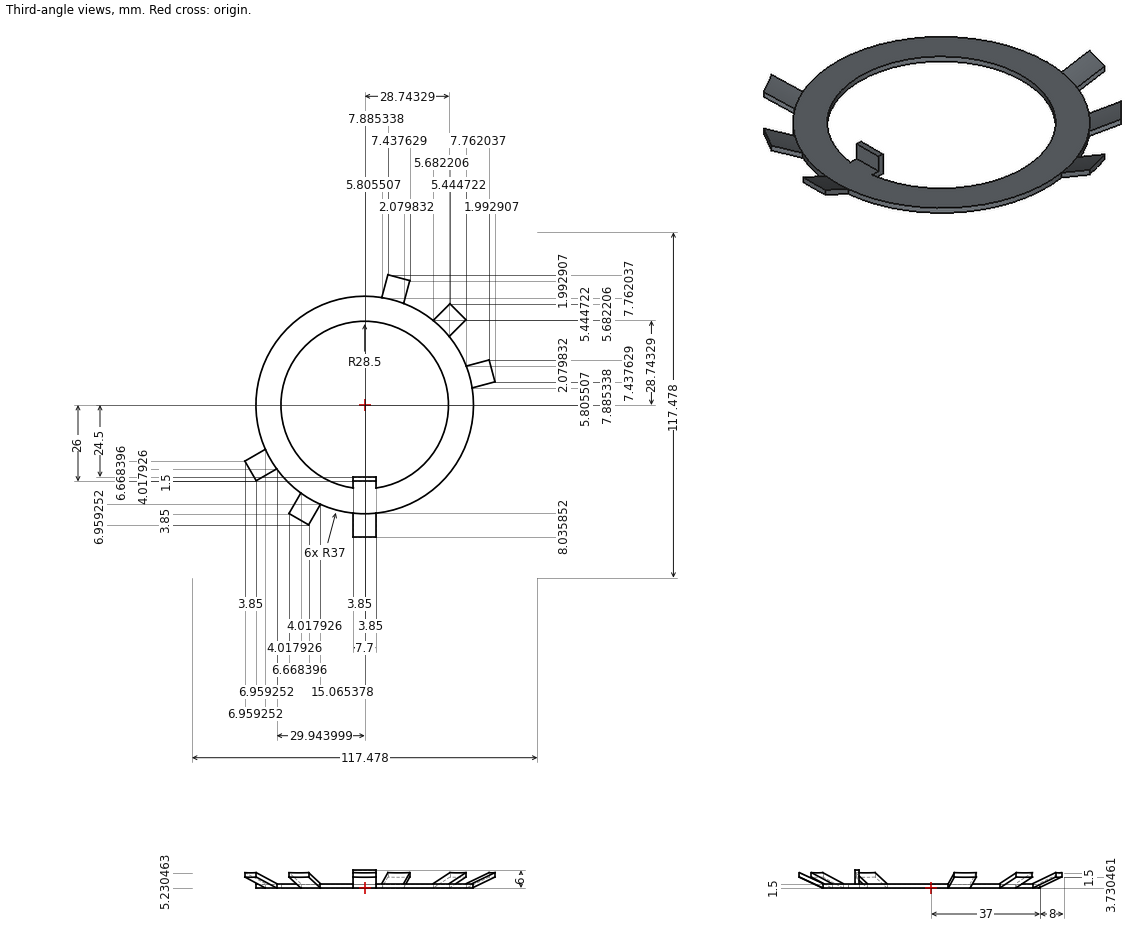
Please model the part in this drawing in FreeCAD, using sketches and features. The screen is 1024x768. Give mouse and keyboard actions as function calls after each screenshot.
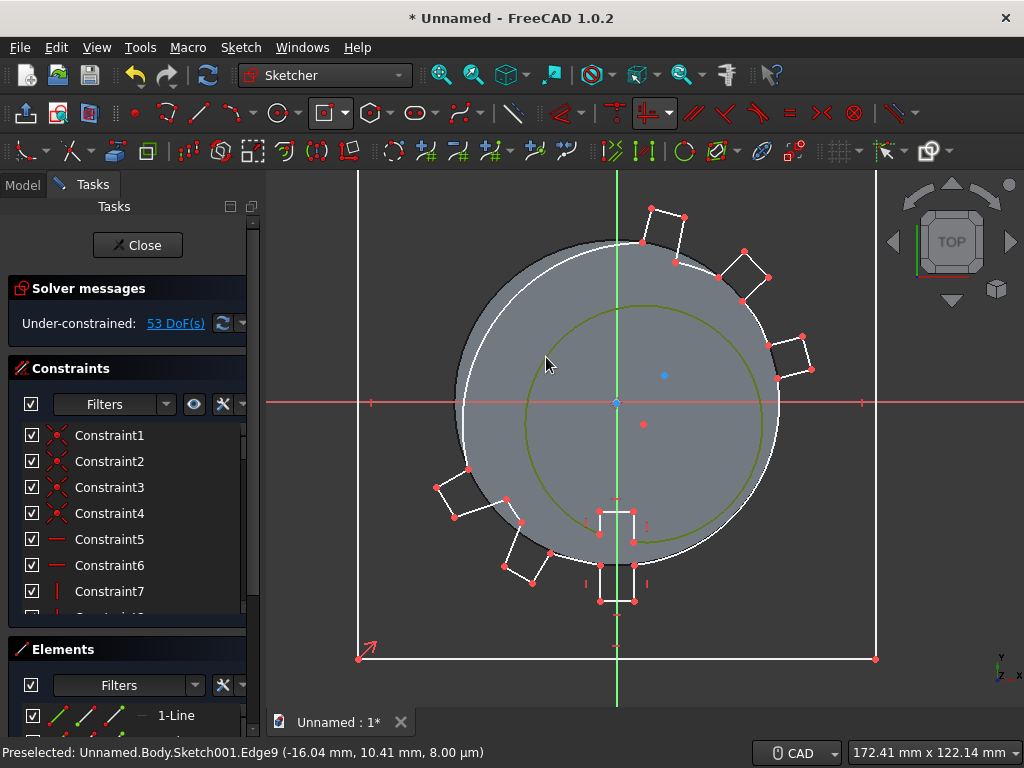
click(763, 331)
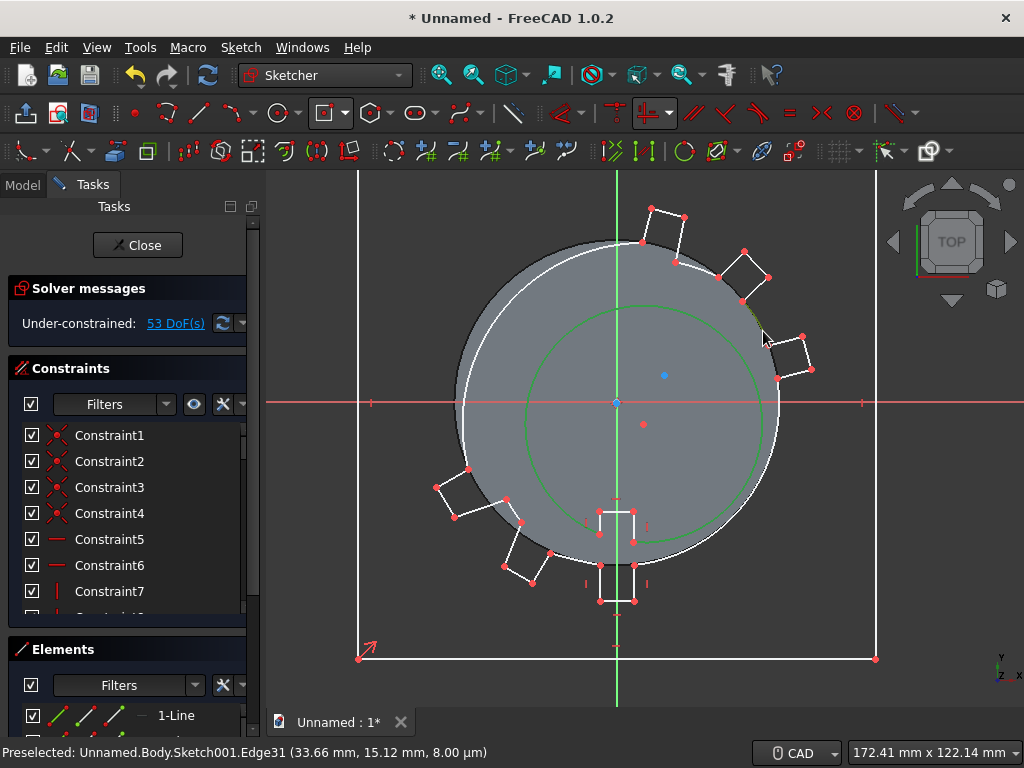
click(616, 114)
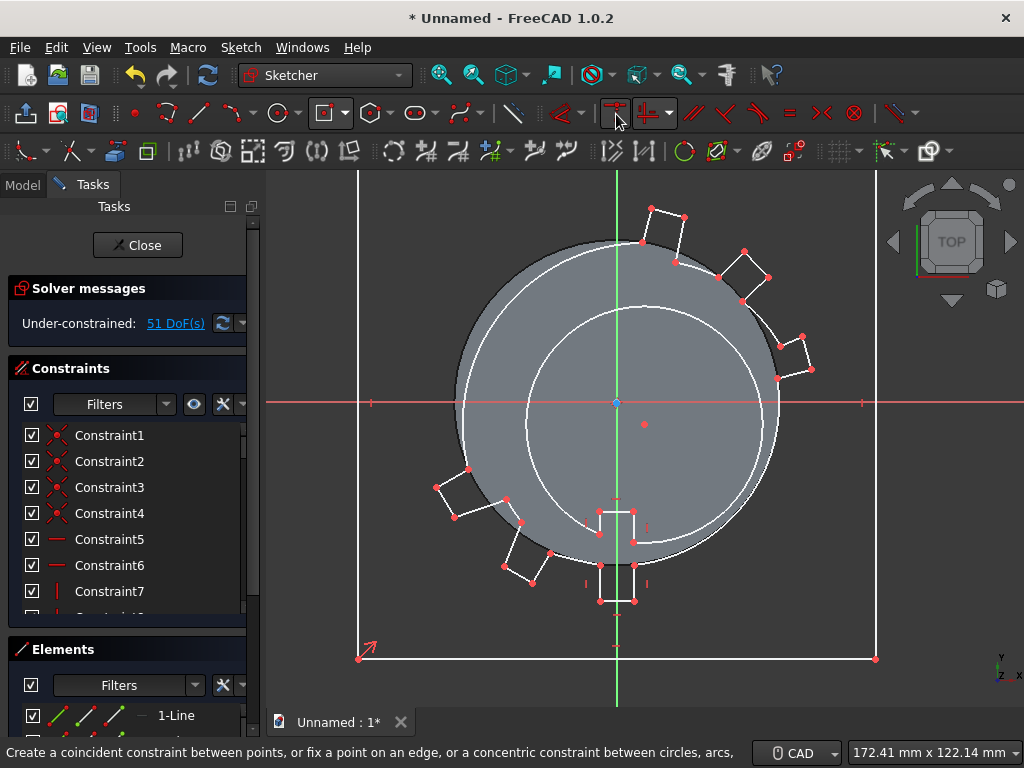
click(548, 357)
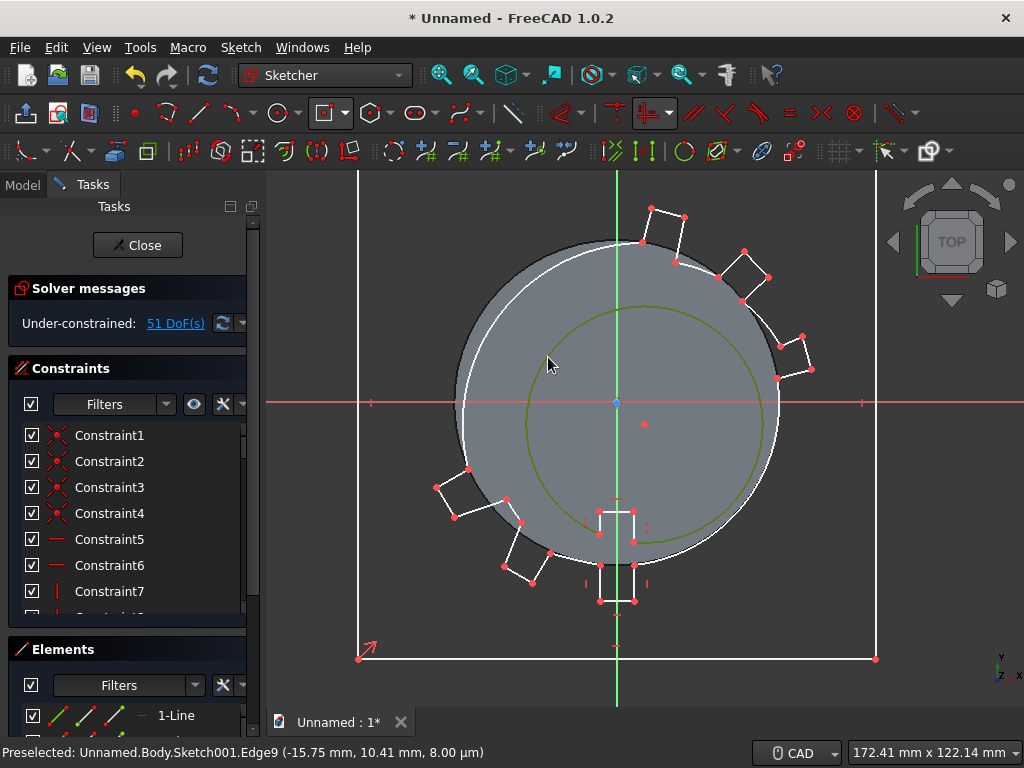
click(707, 538)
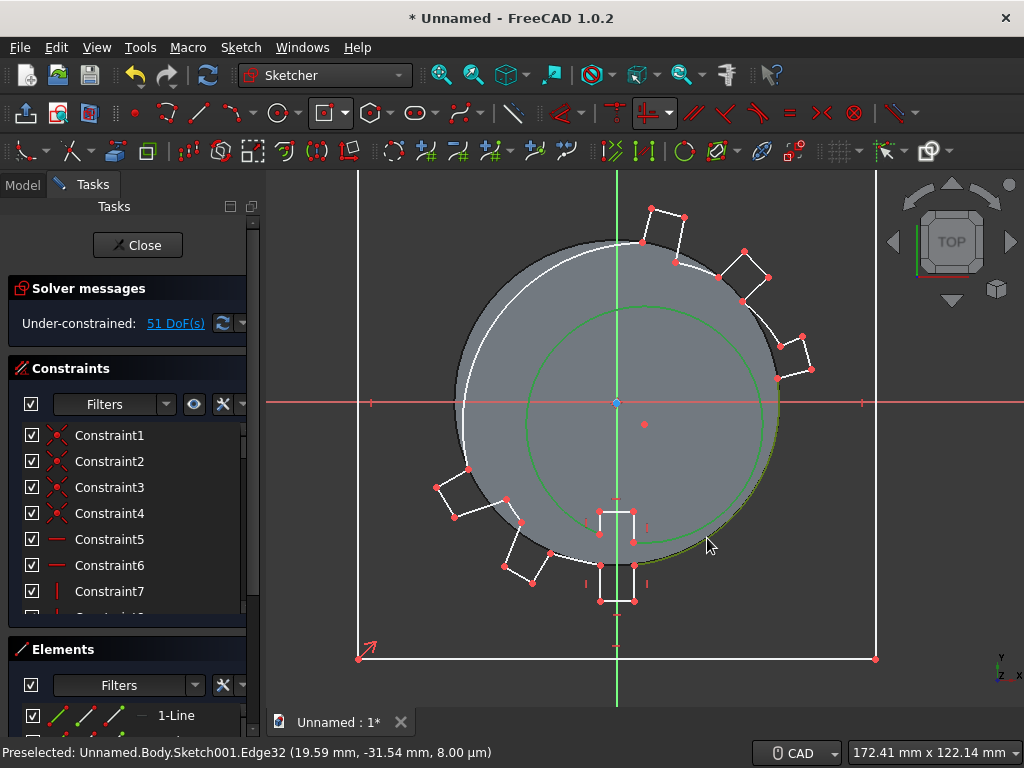
key(c)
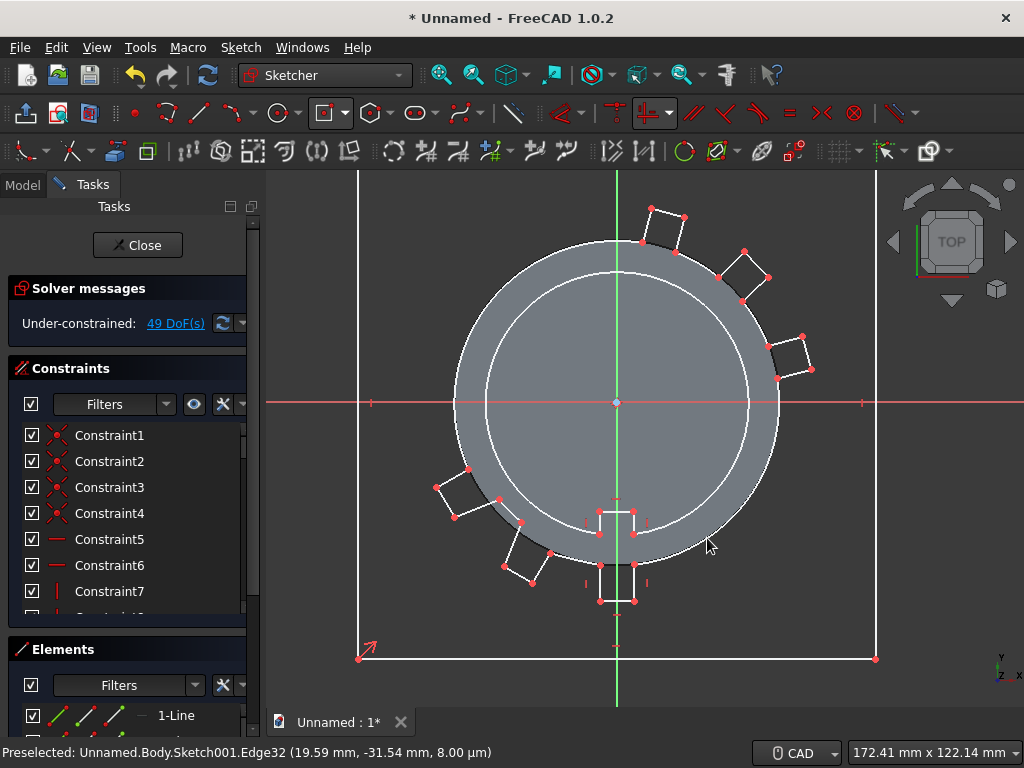
click(740, 357)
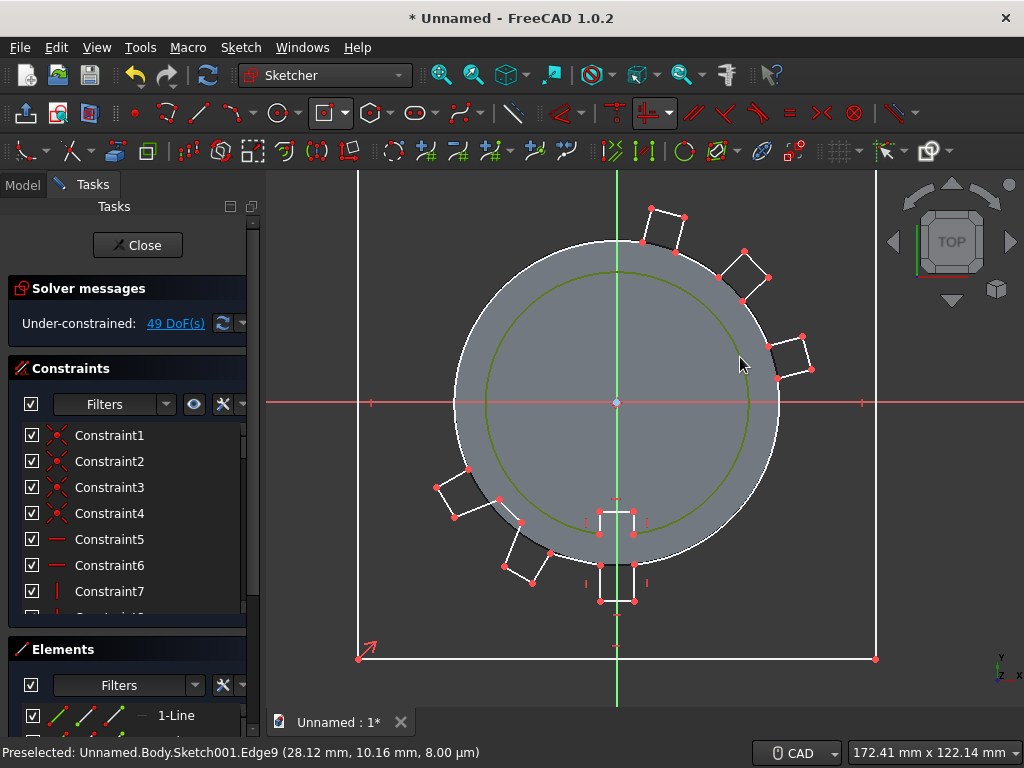
click(565, 557)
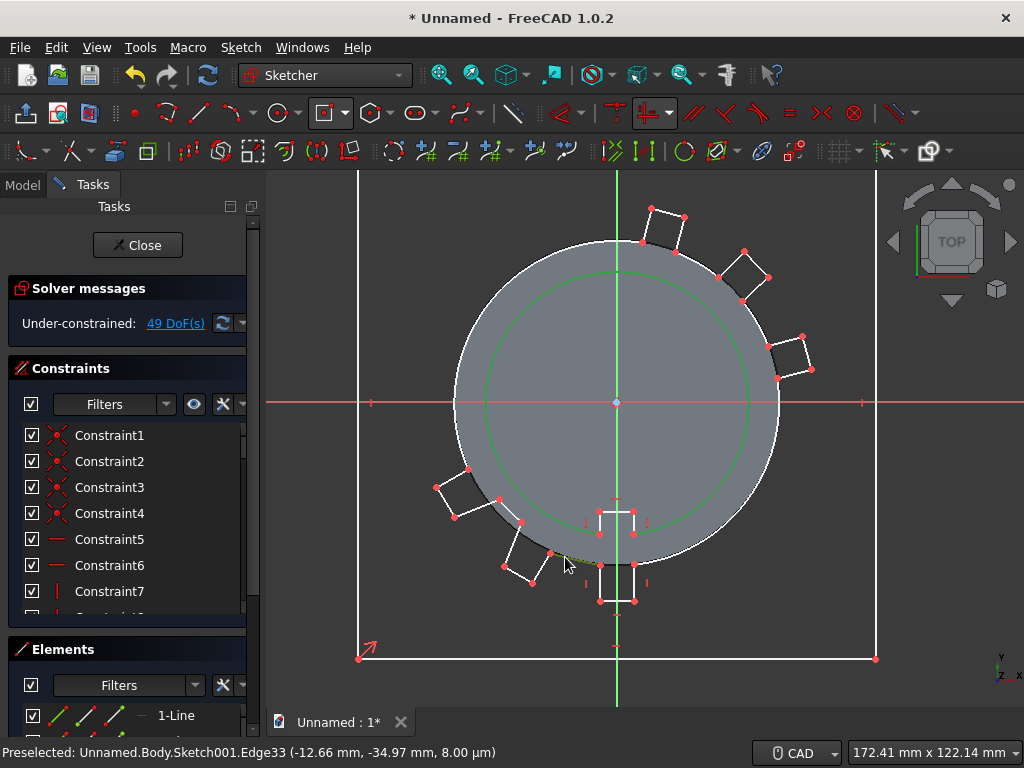
click(616, 114)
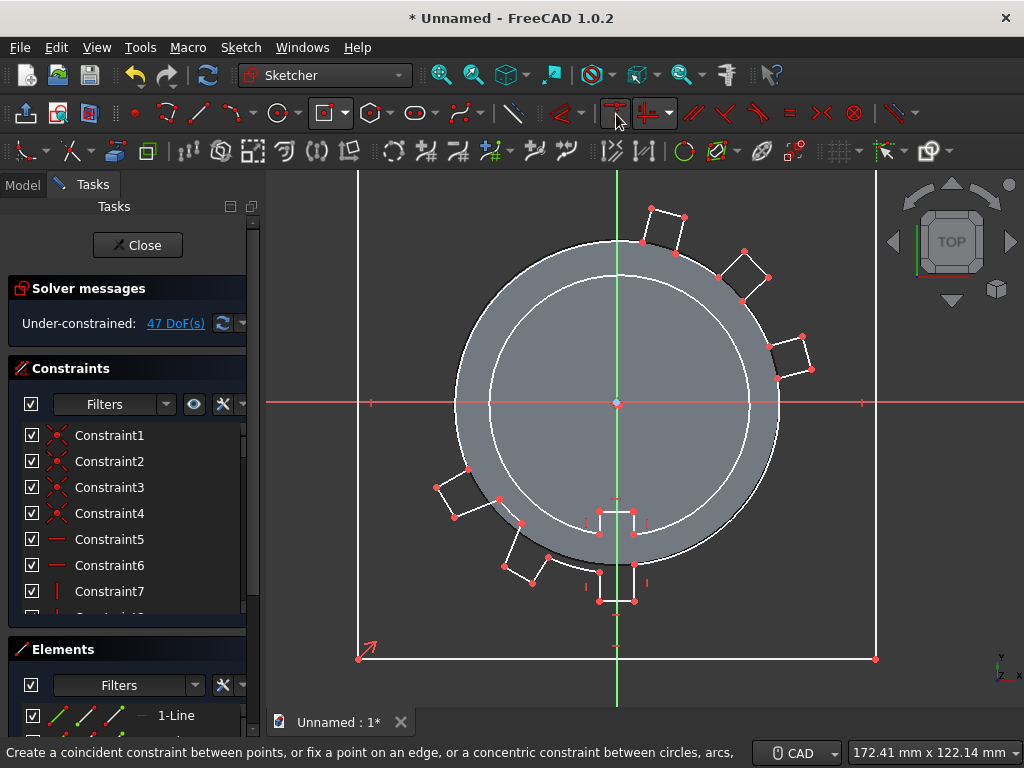
drag(607, 392, 630, 415)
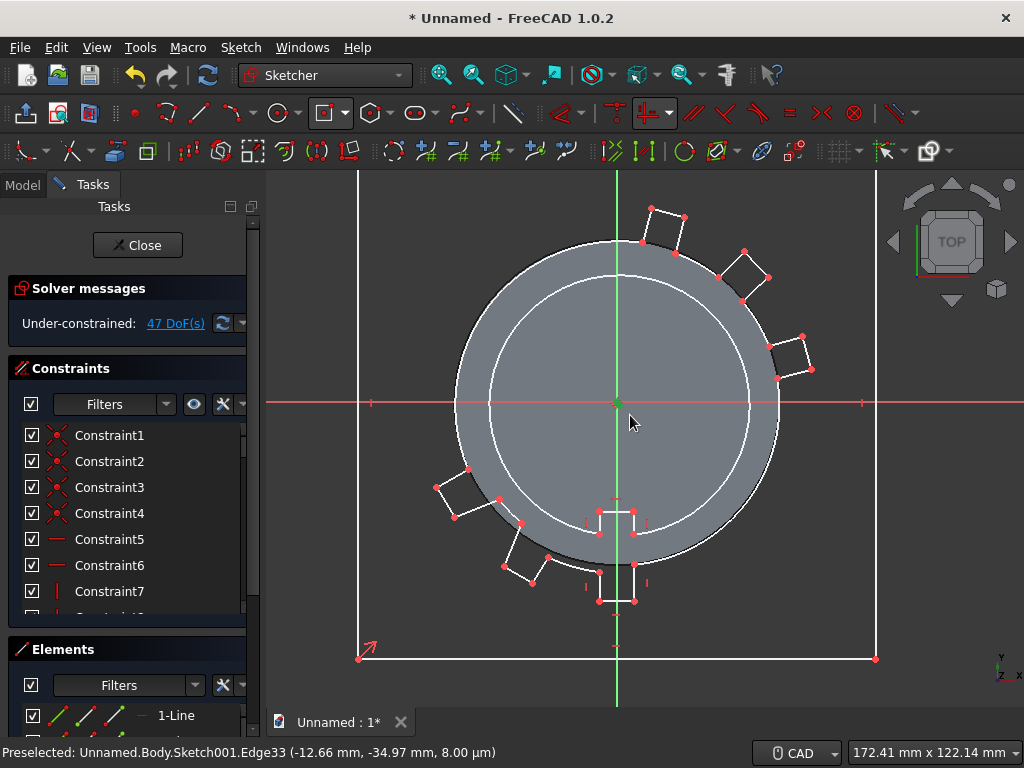
click(616, 114)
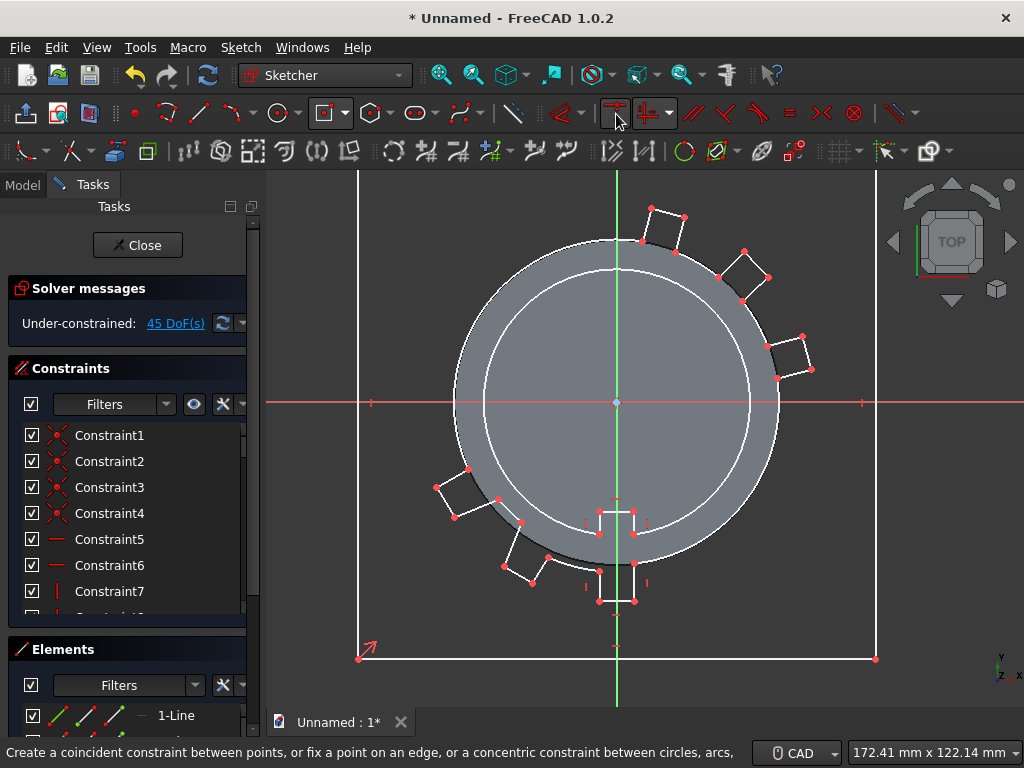
scroll(505, 507, up, 2)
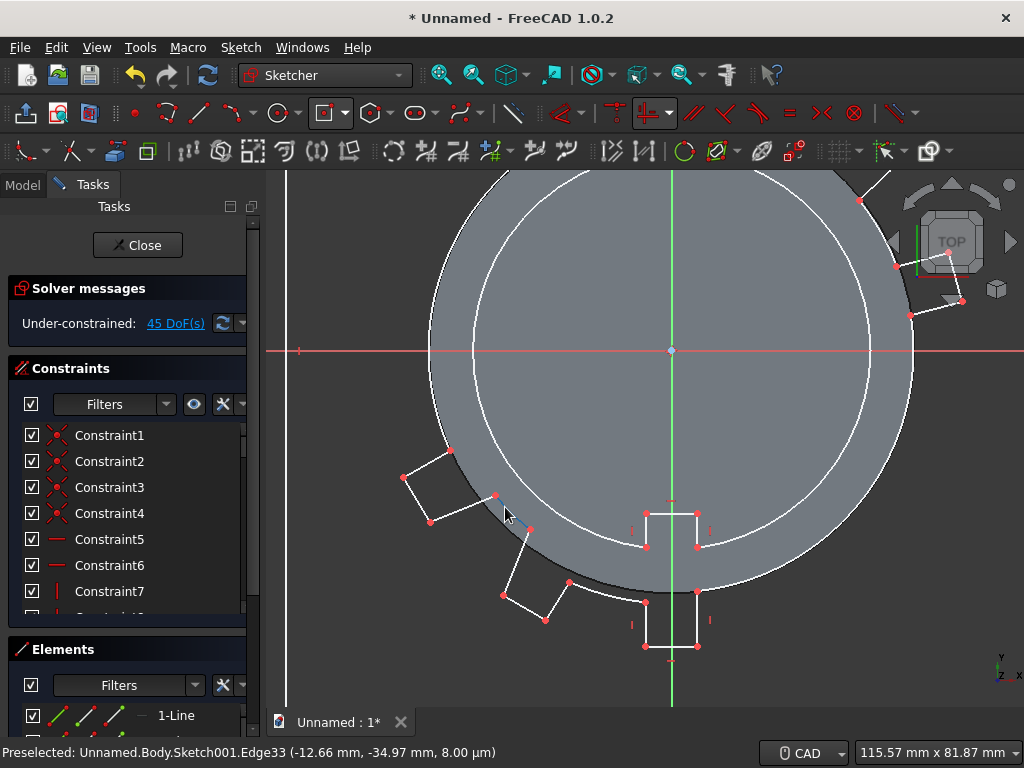
click(505, 507)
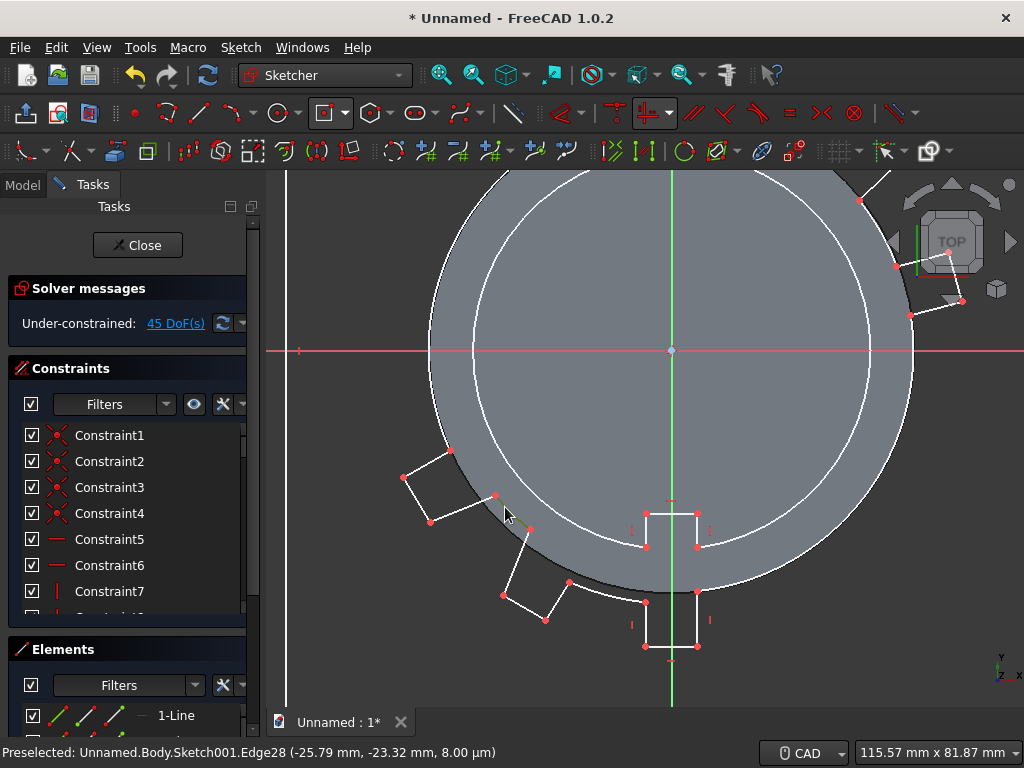
click(435, 297)